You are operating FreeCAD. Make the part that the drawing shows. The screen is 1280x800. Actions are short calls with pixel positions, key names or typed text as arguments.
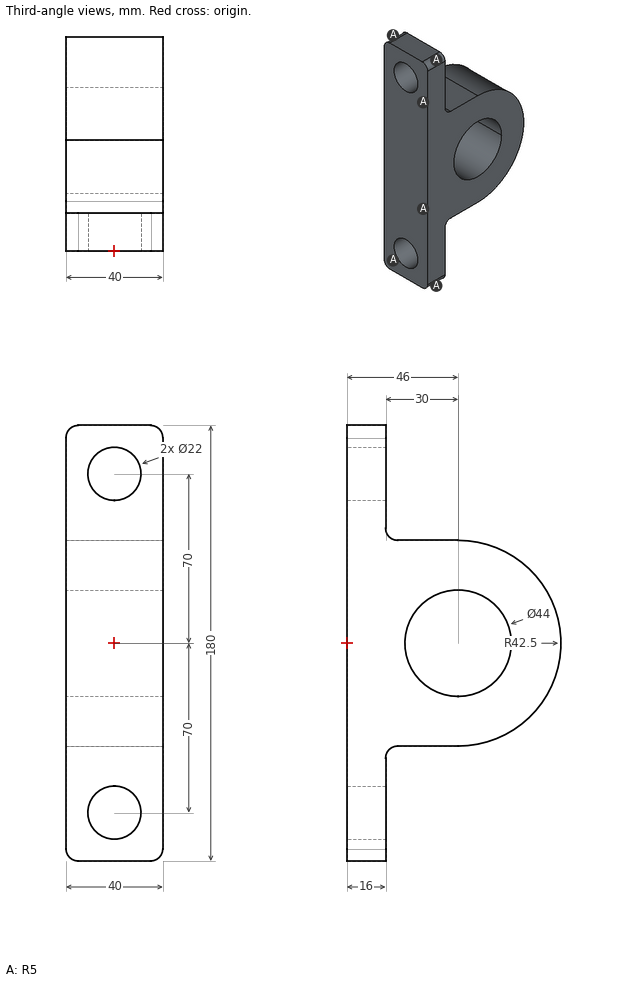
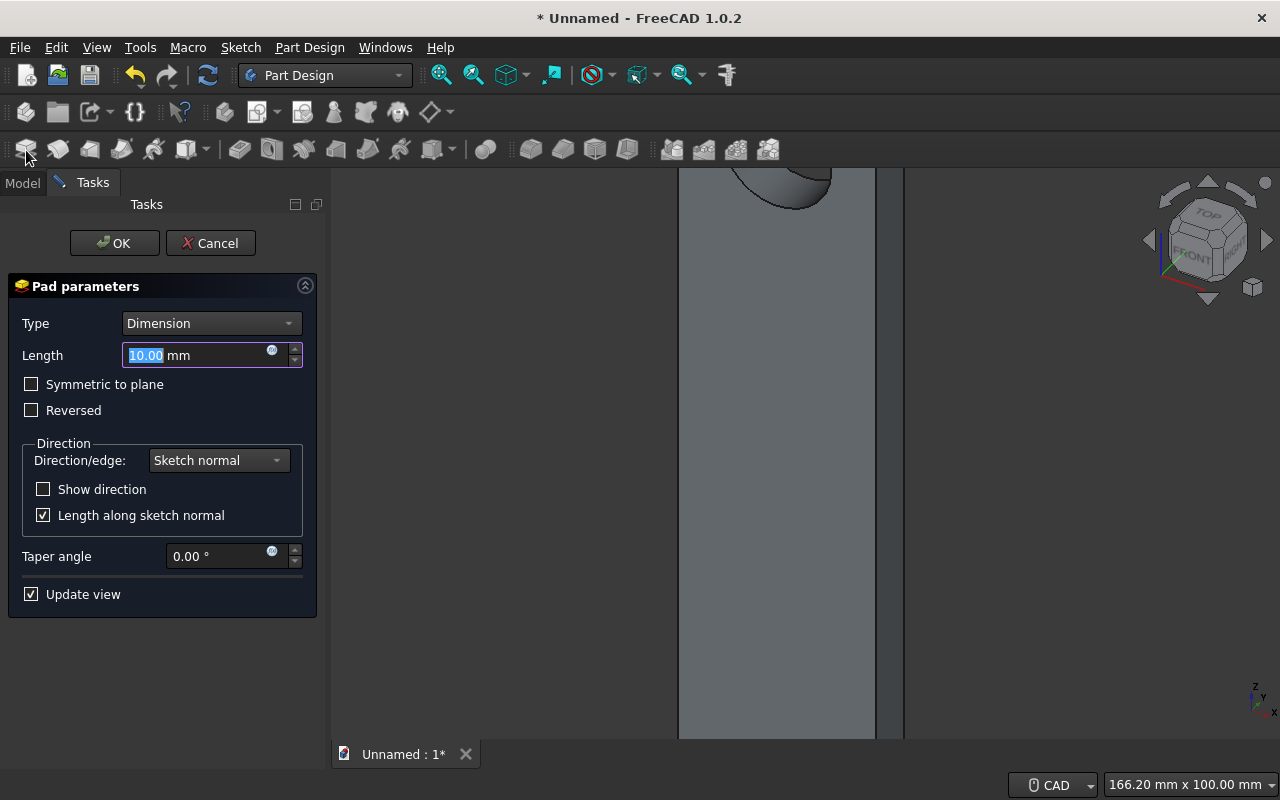
text(16)
key(Tab)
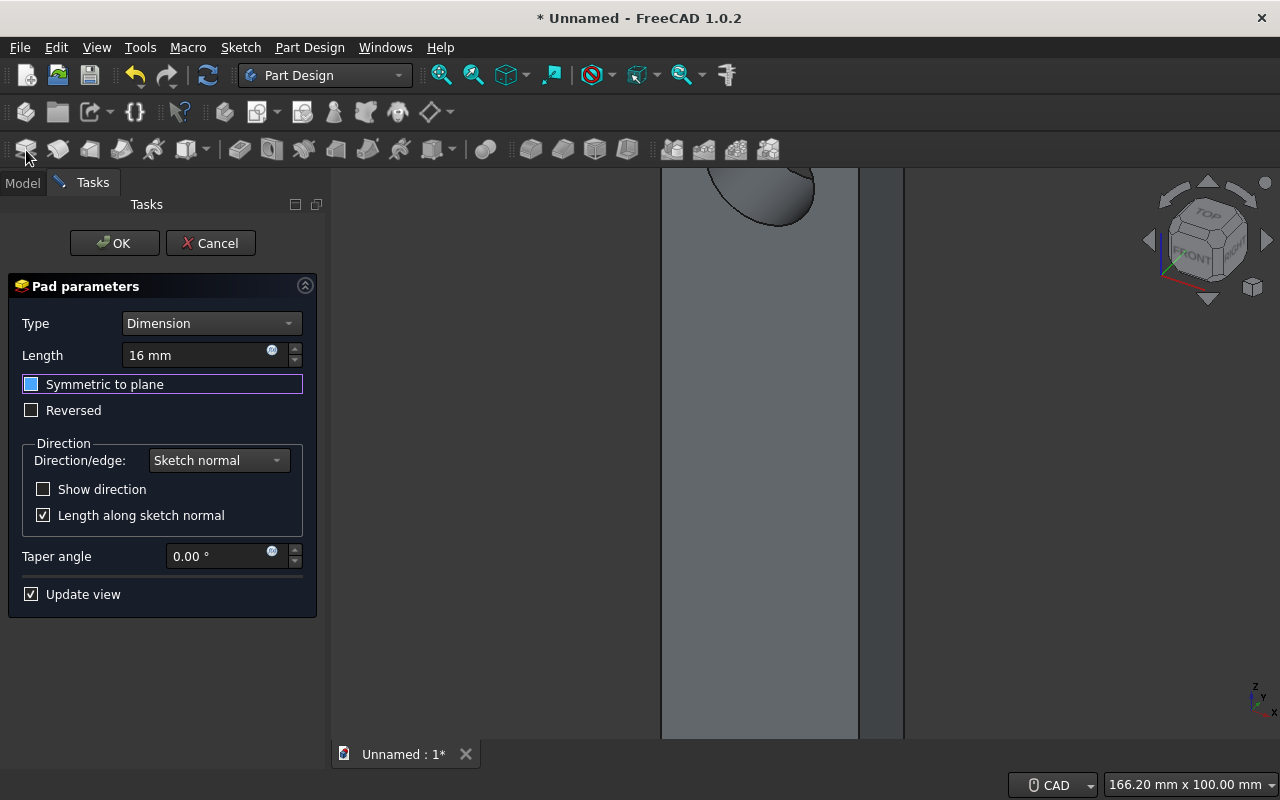
click(30, 410)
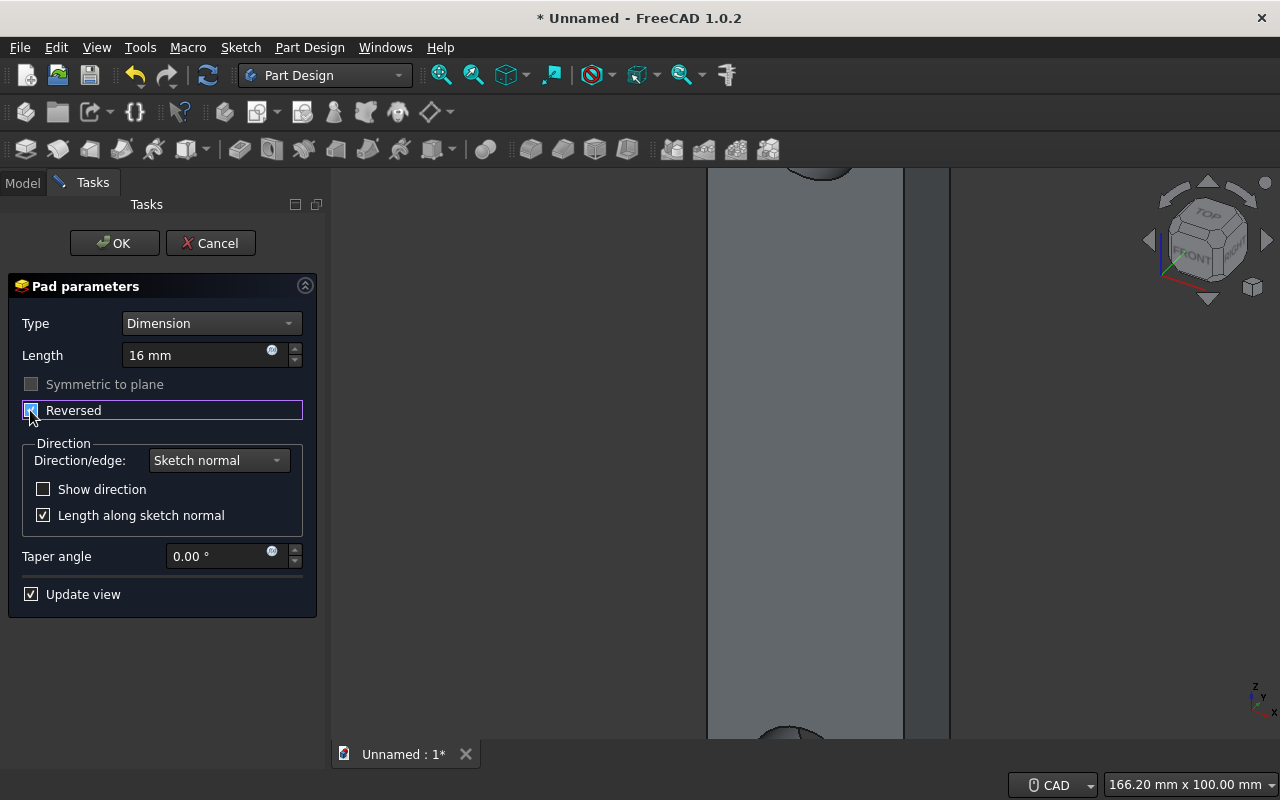
click(115, 243)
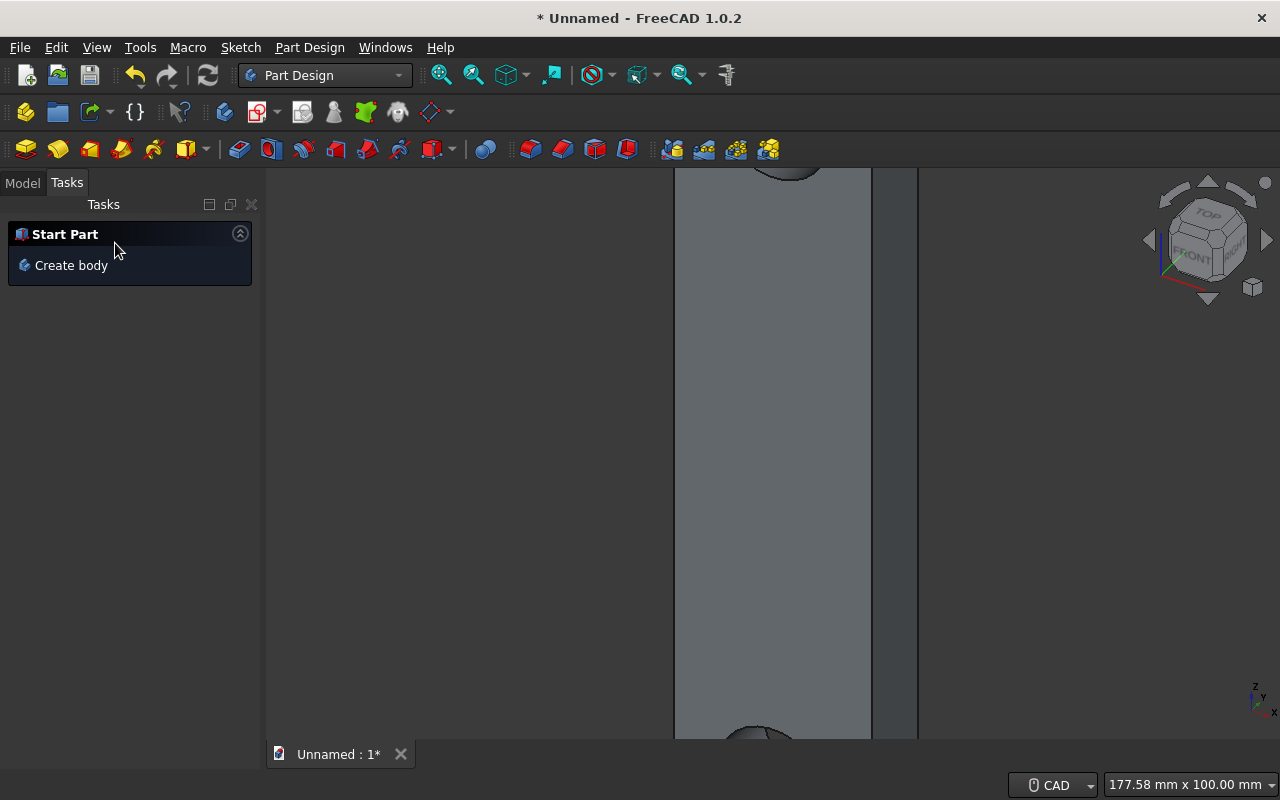
key(v)
key(f)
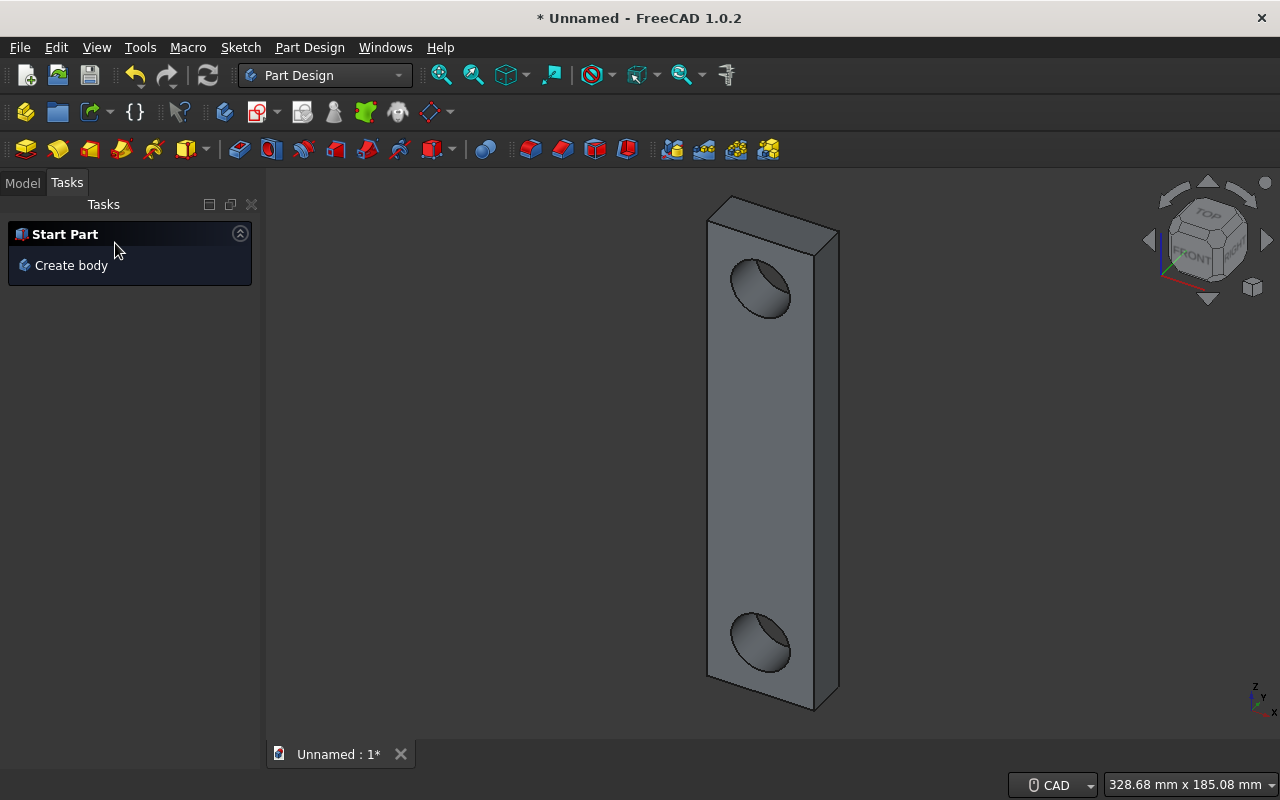
click(258, 112)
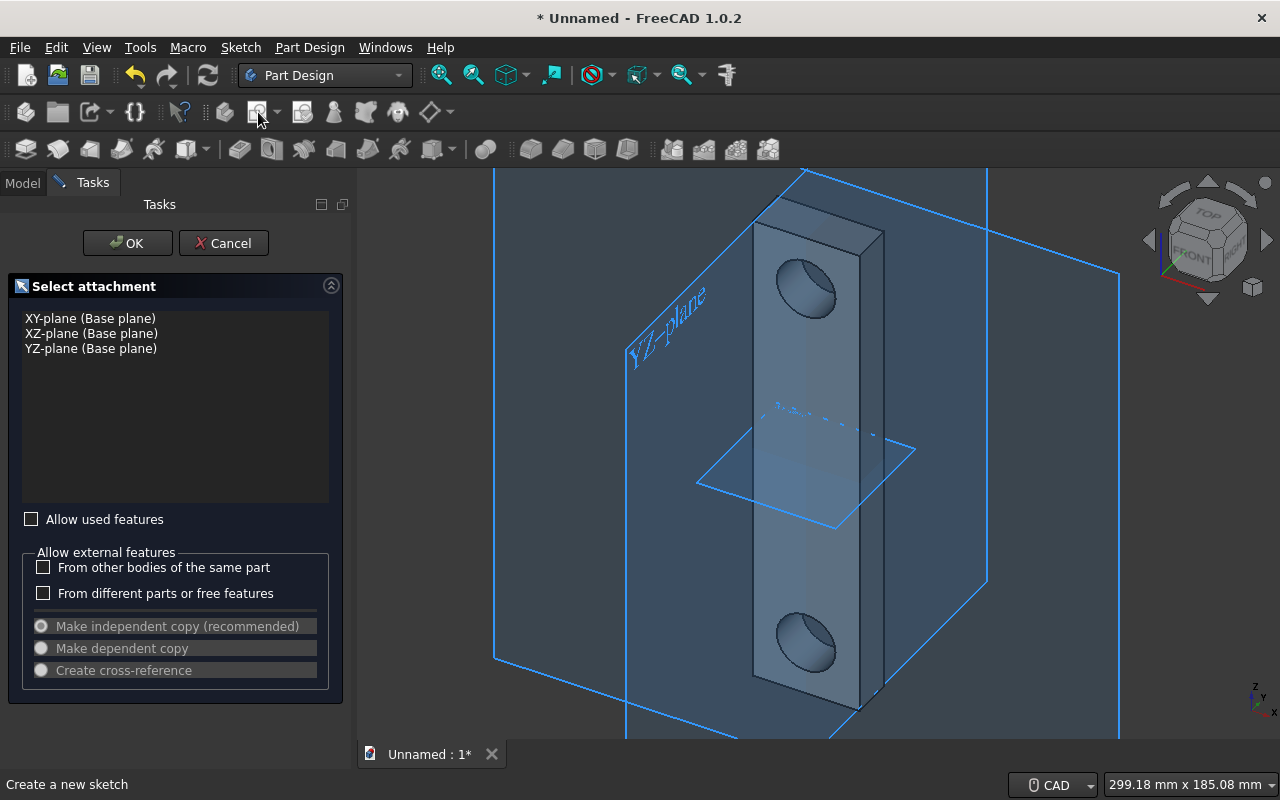
click(82, 348)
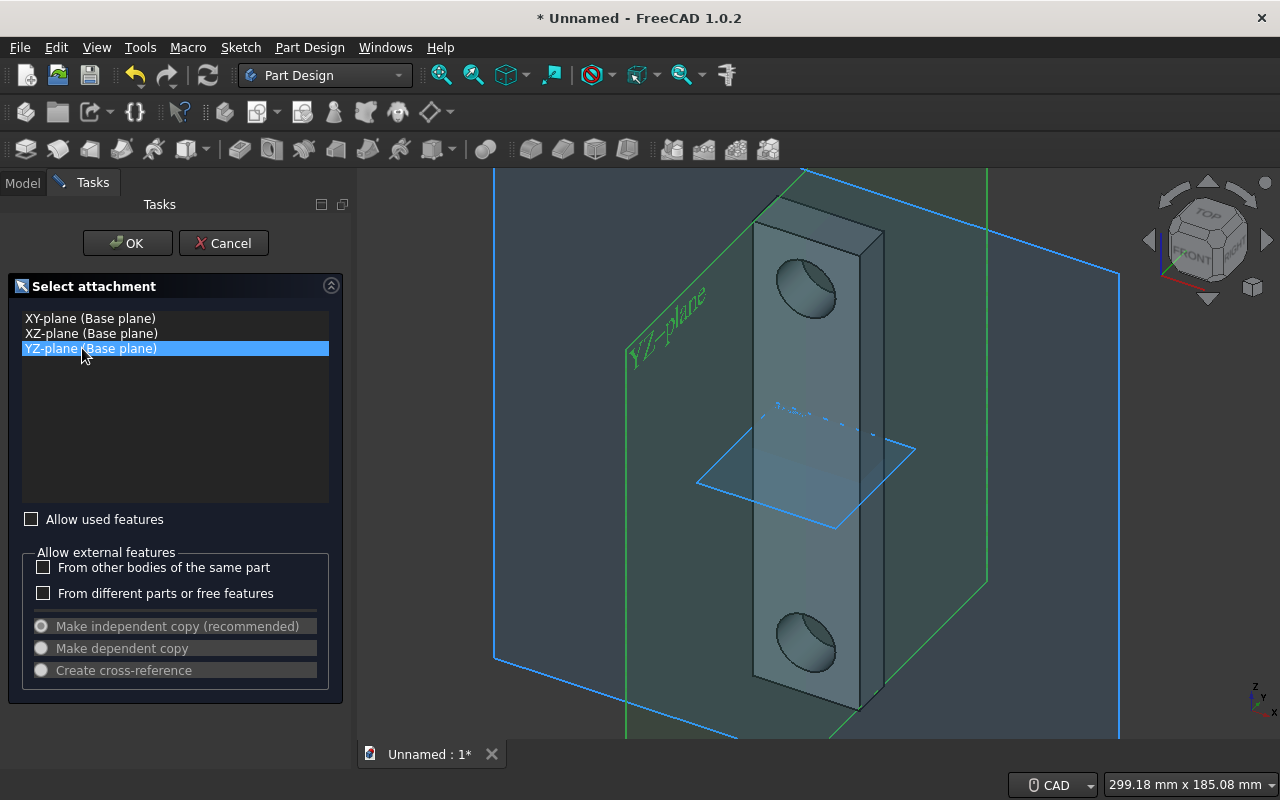
click(128, 243)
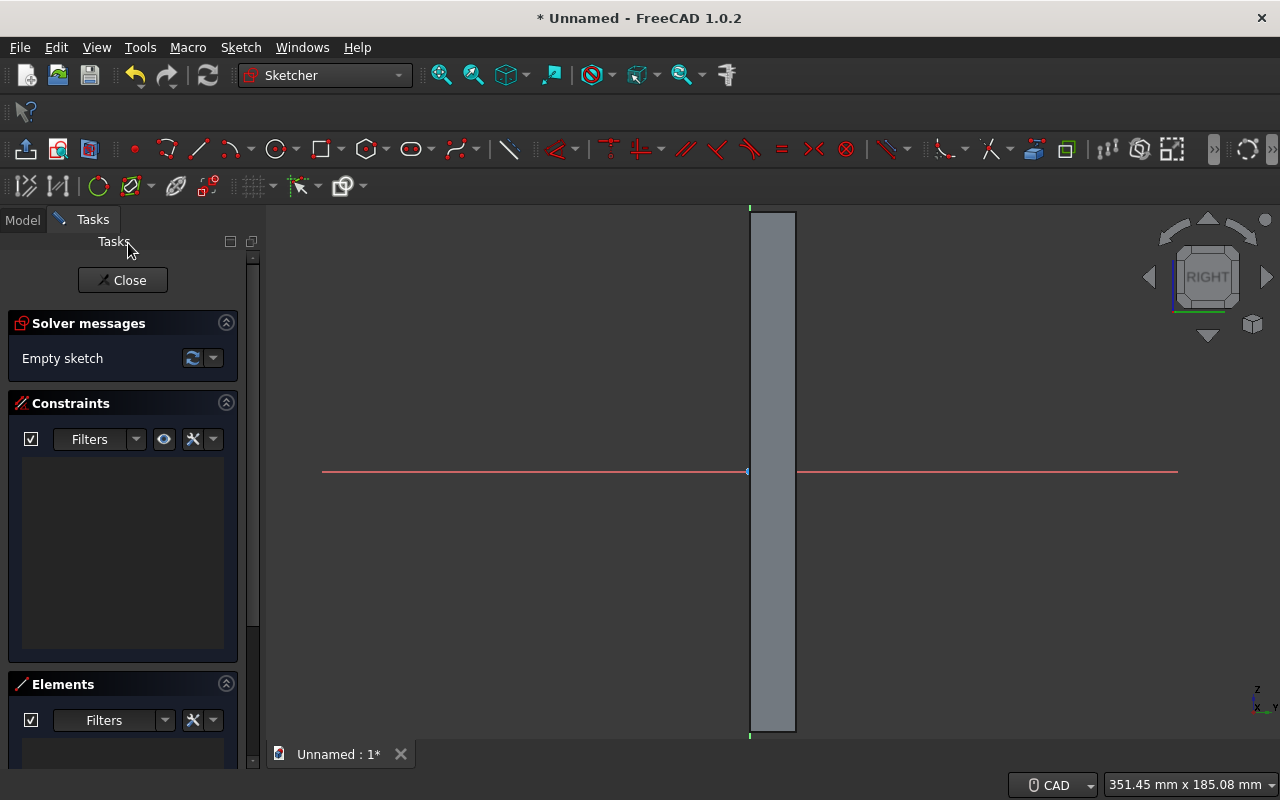
click(90, 150)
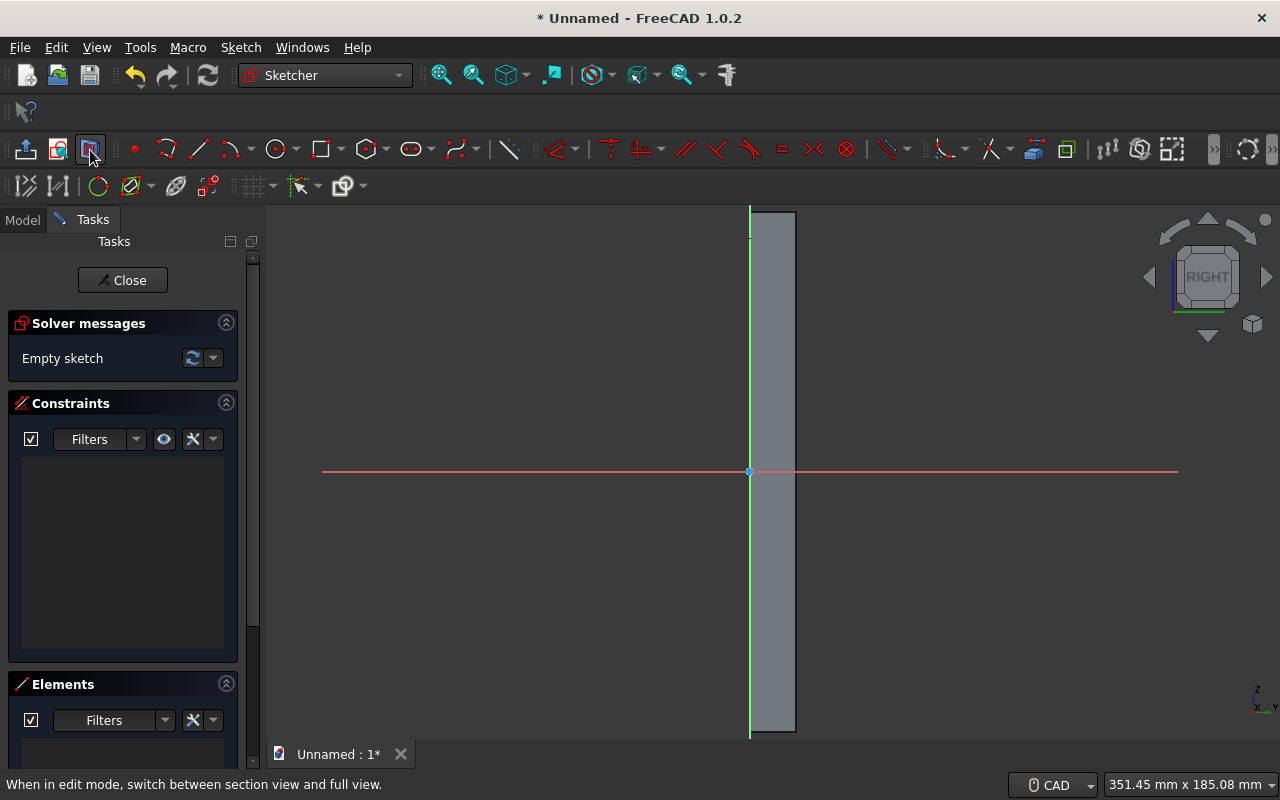
scroll(1115, 472, up, 2)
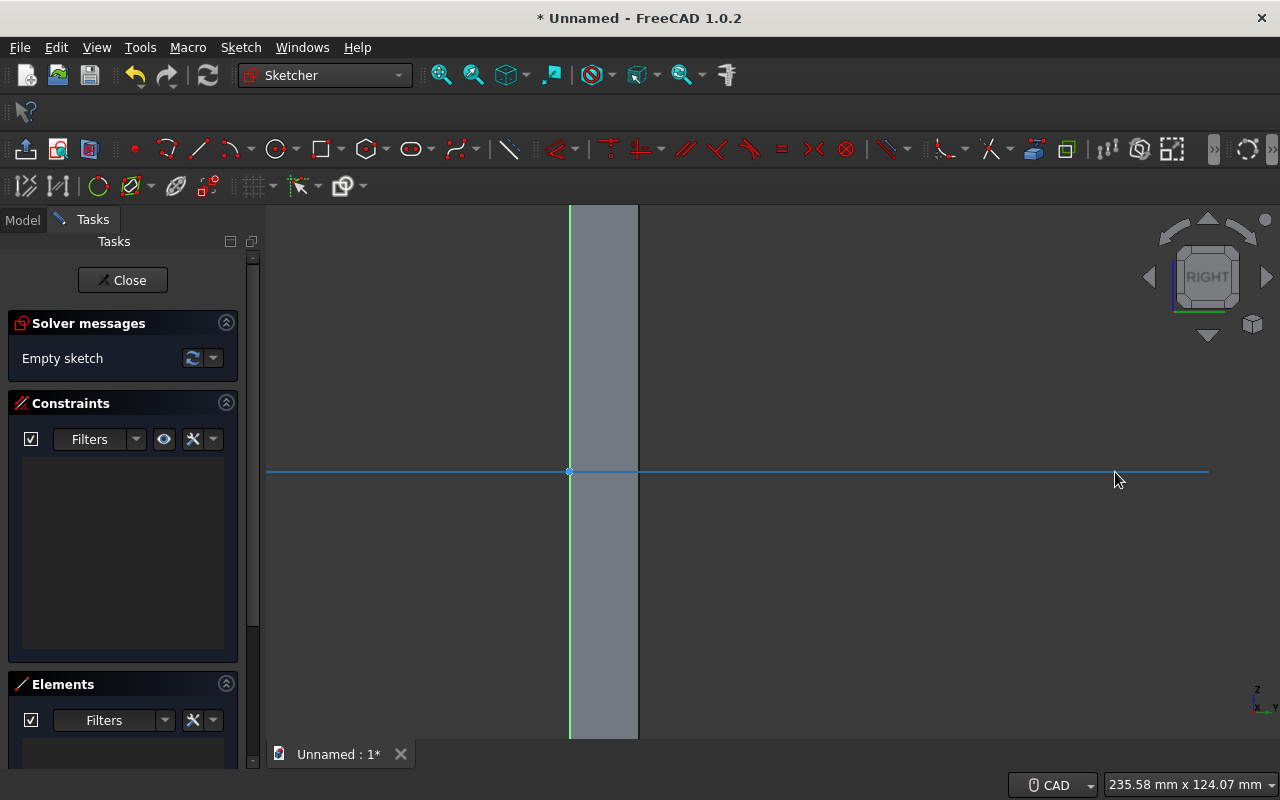
click(168, 150)